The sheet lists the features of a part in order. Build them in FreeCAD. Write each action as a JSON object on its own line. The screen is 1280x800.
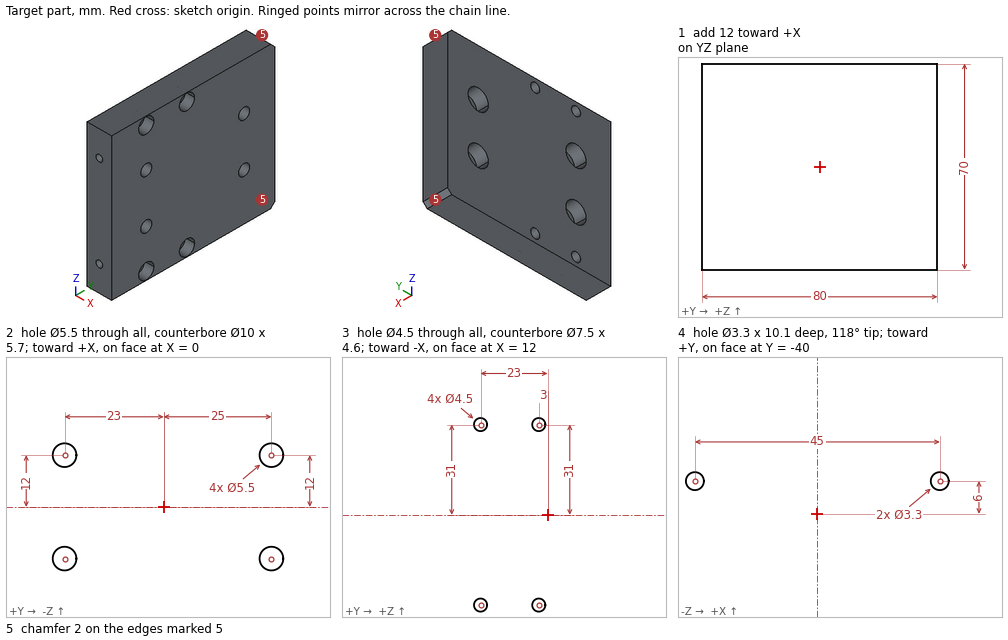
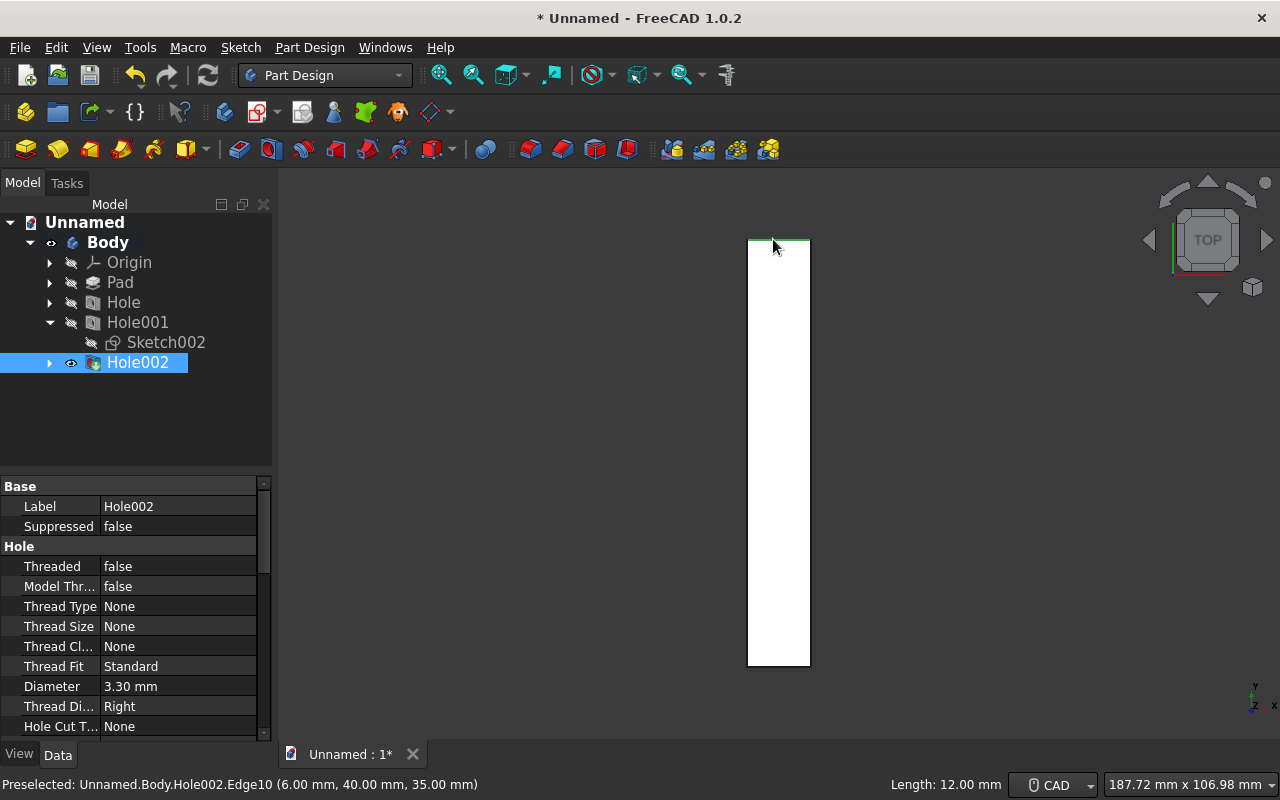
{"action": "key", "text": "0"}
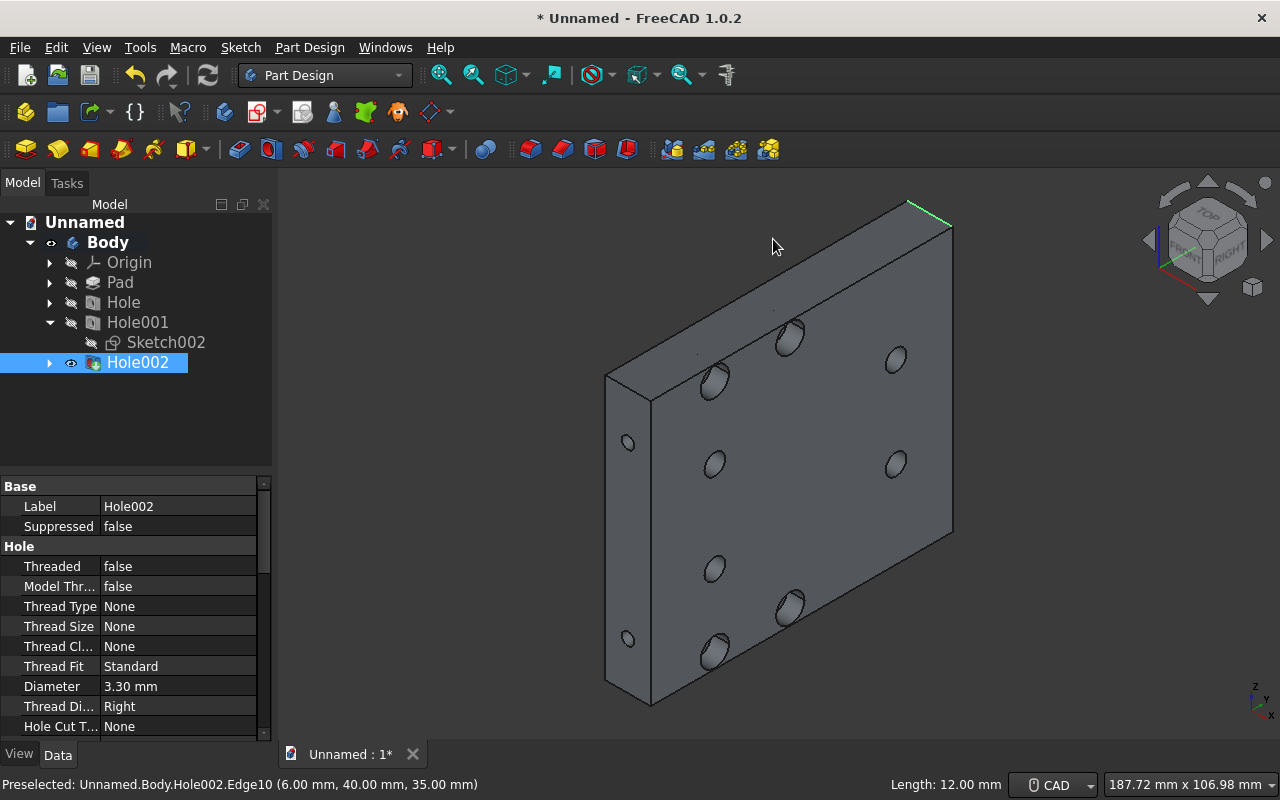
{"action": "key", "text": "1"}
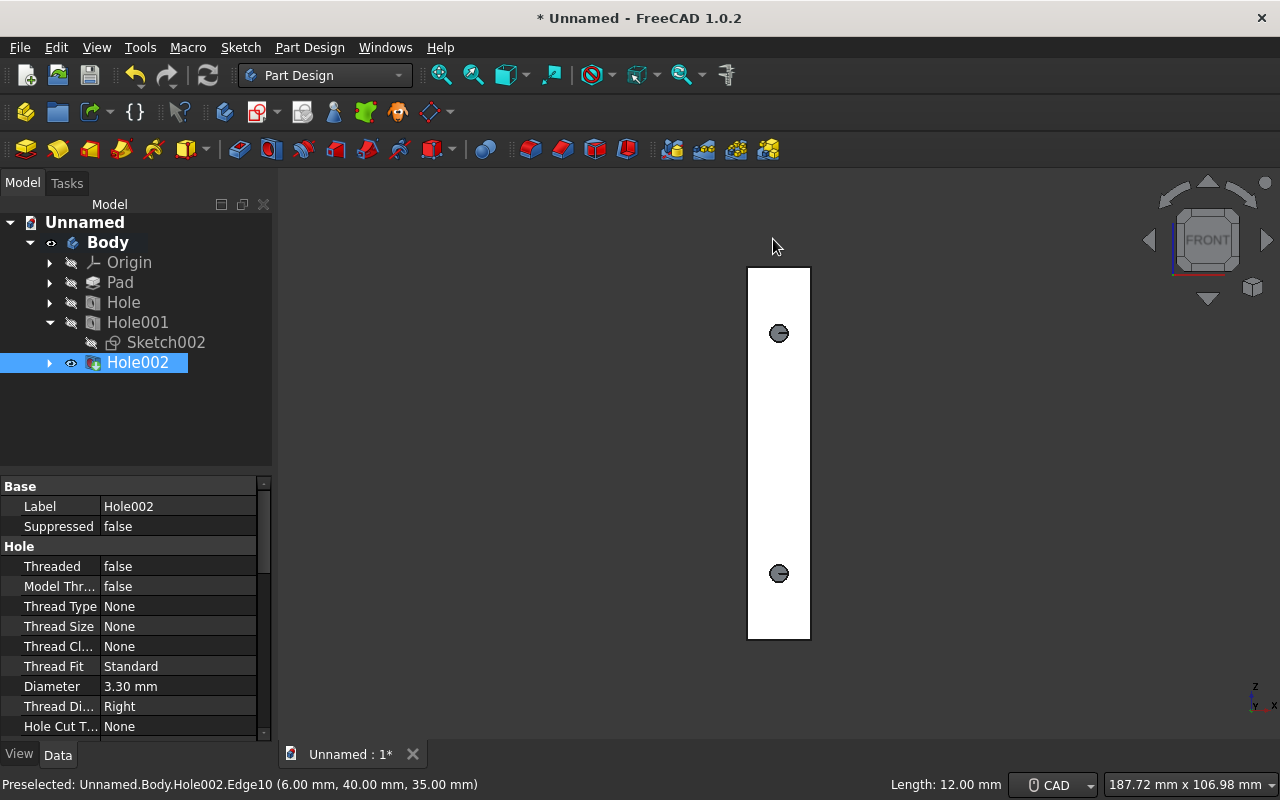
{"action": "key", "text": "3"}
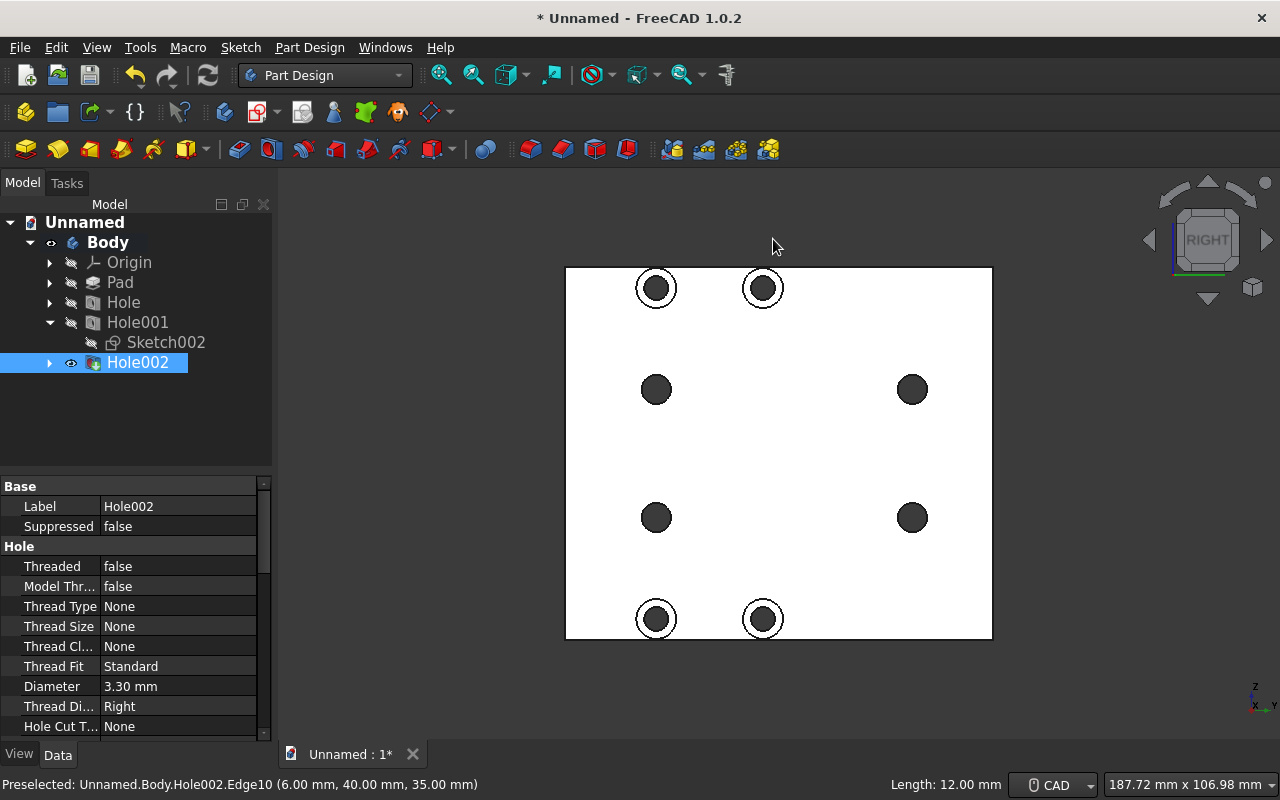
{"action": "key", "text": "5"}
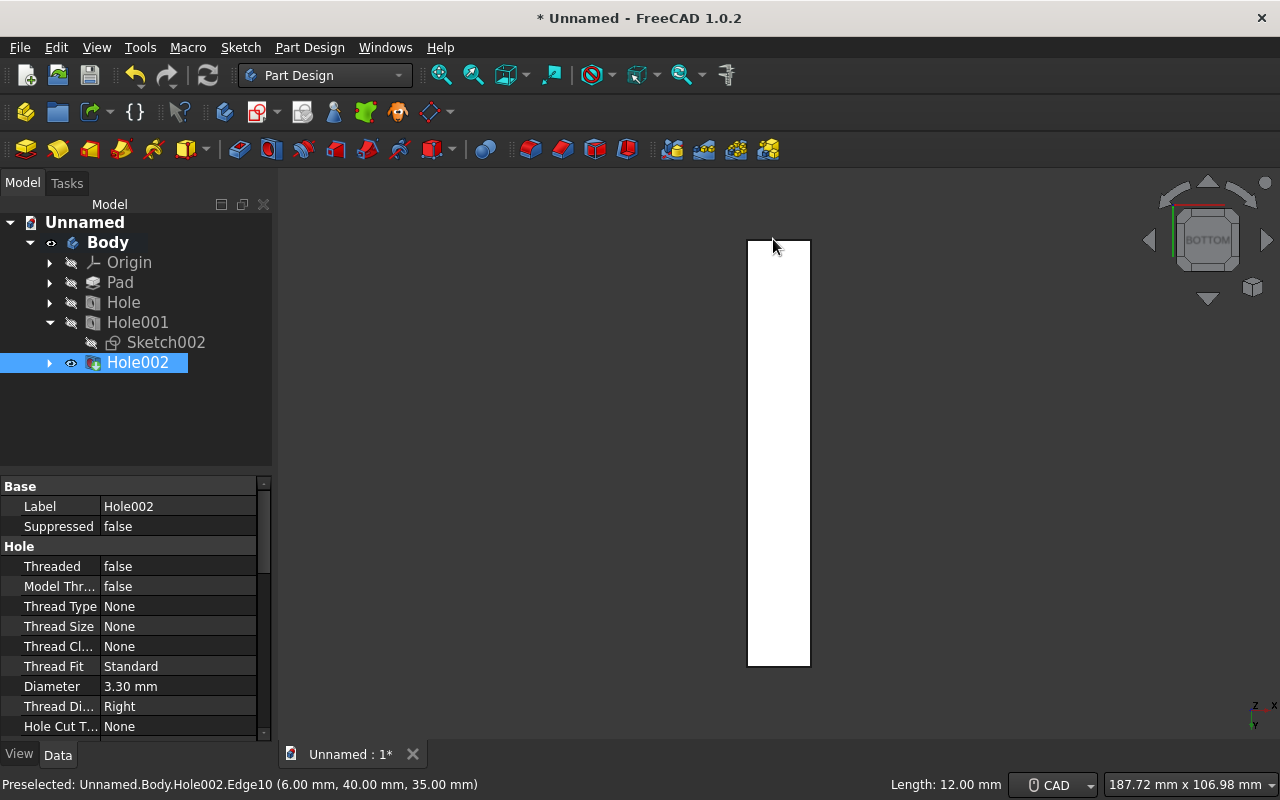
{"action": "left_click", "coordinate": [779, 666], "text": "ctrl"}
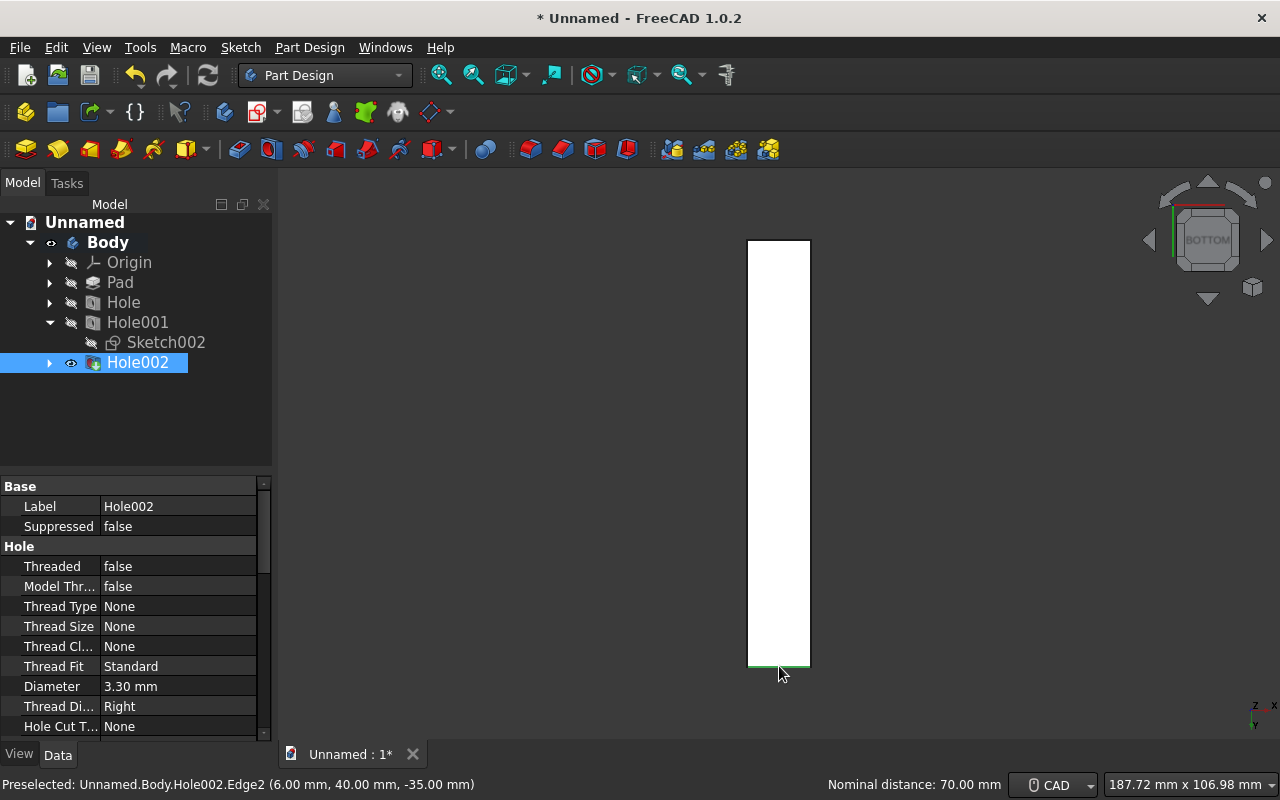
{"action": "left_click", "coordinate": [564, 150]}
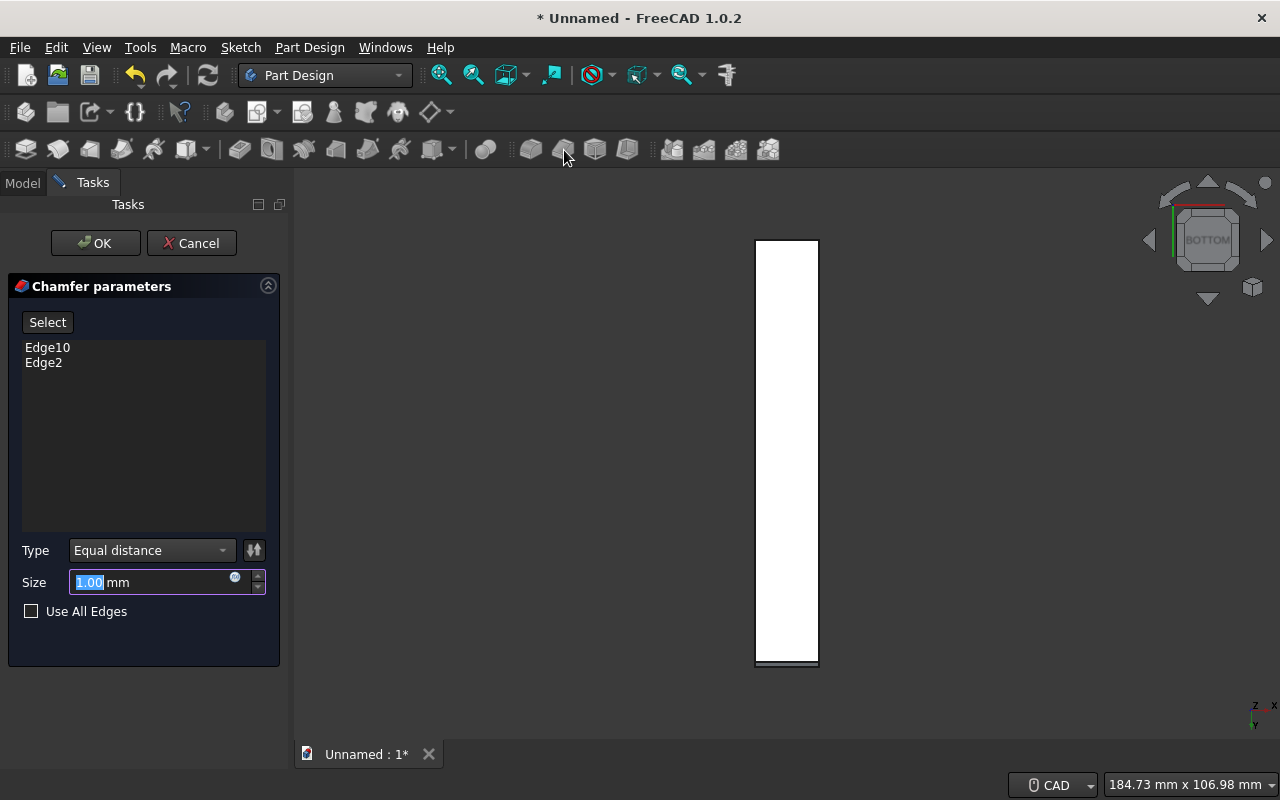
{"action": "type", "text": "2"}
{"action": "key", "text": "Tab"}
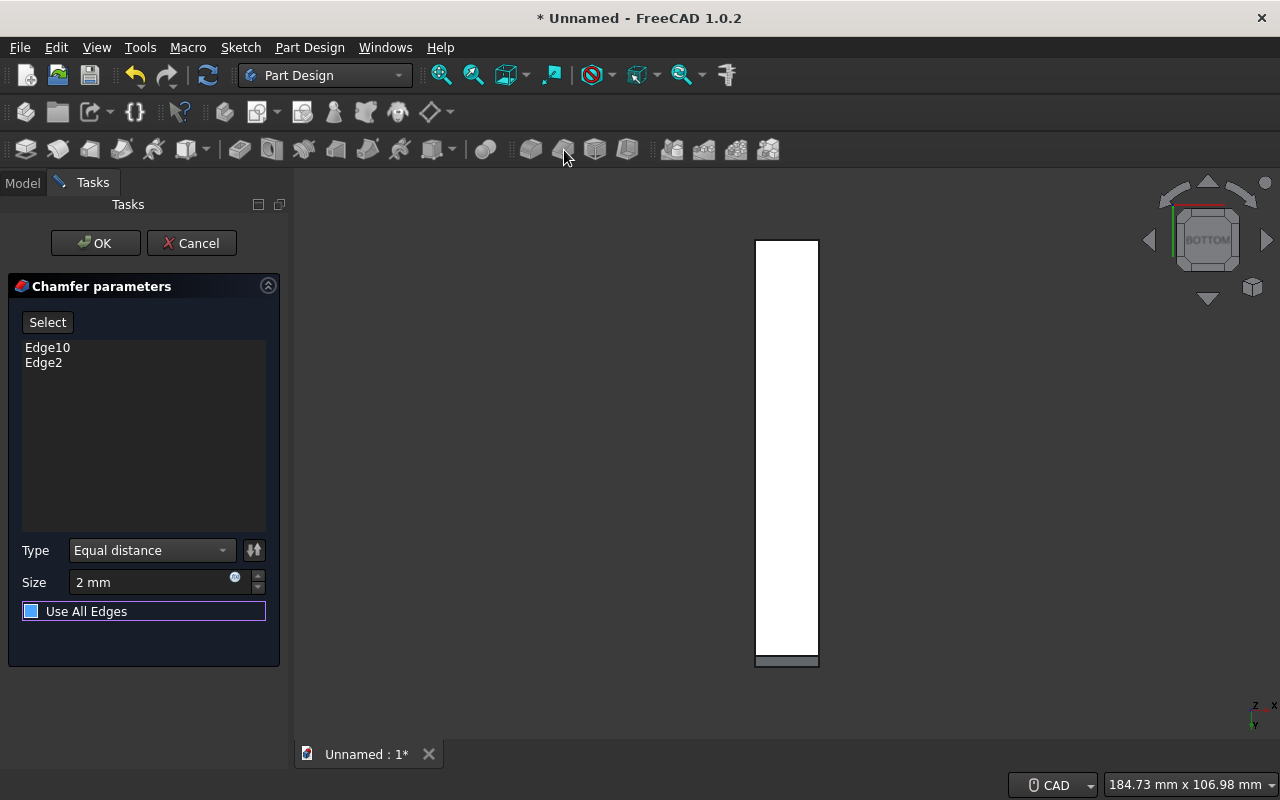
{"action": "left_click", "coordinate": [96, 243]}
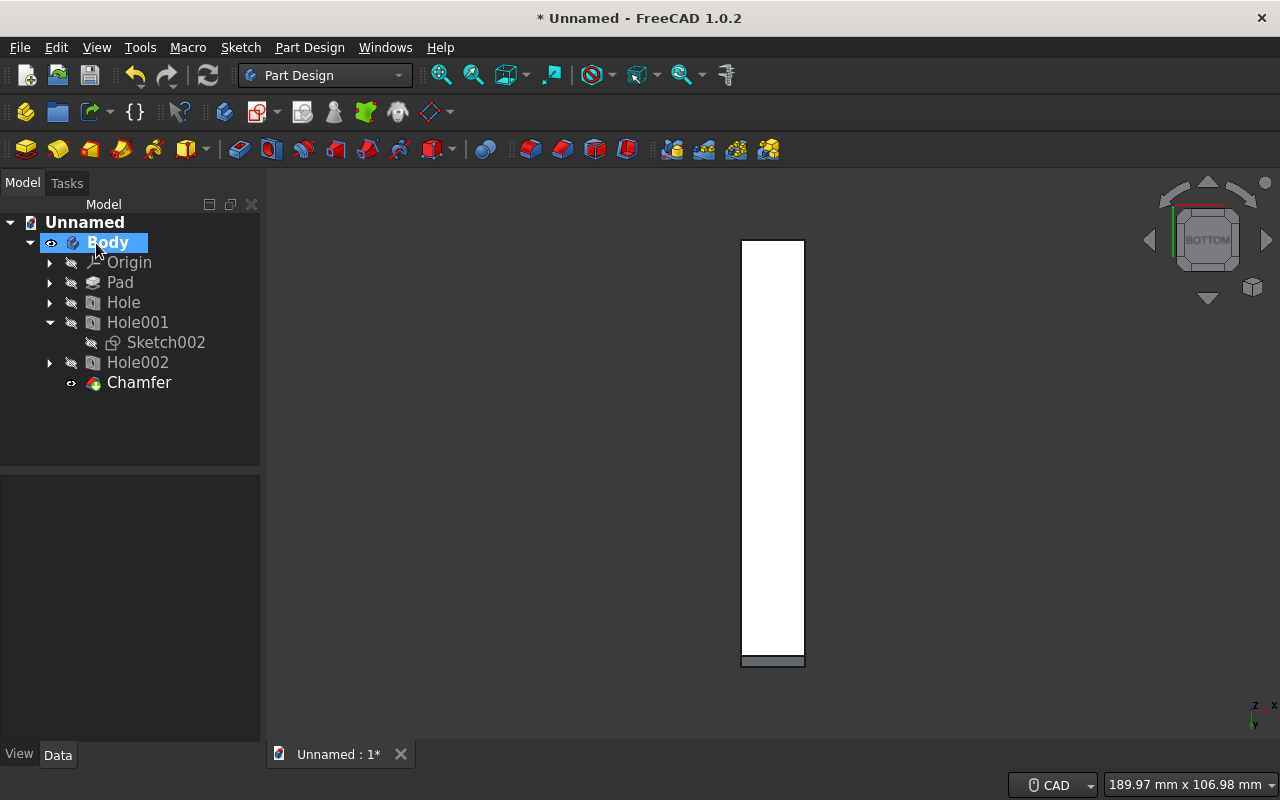
{"action": "key", "text": "0"}